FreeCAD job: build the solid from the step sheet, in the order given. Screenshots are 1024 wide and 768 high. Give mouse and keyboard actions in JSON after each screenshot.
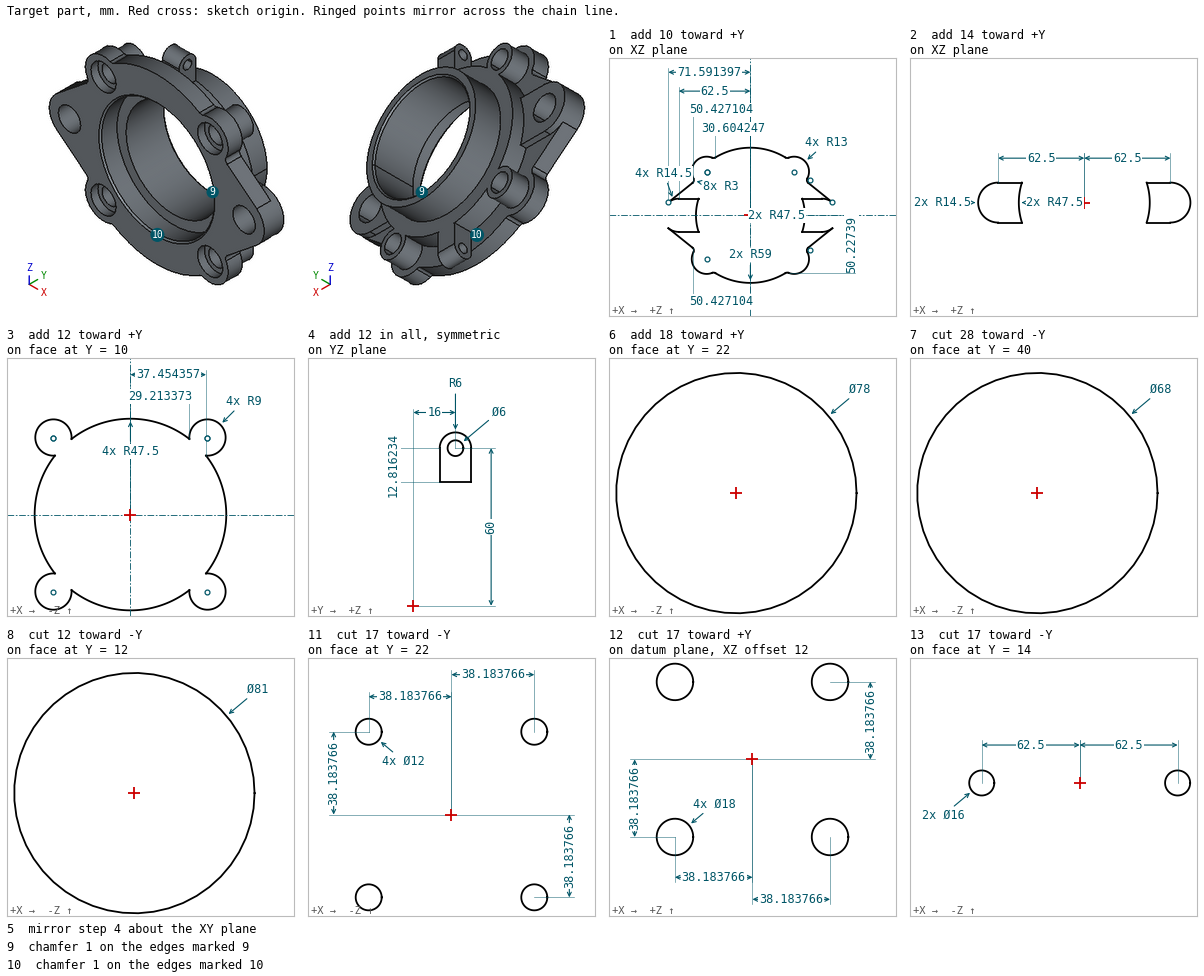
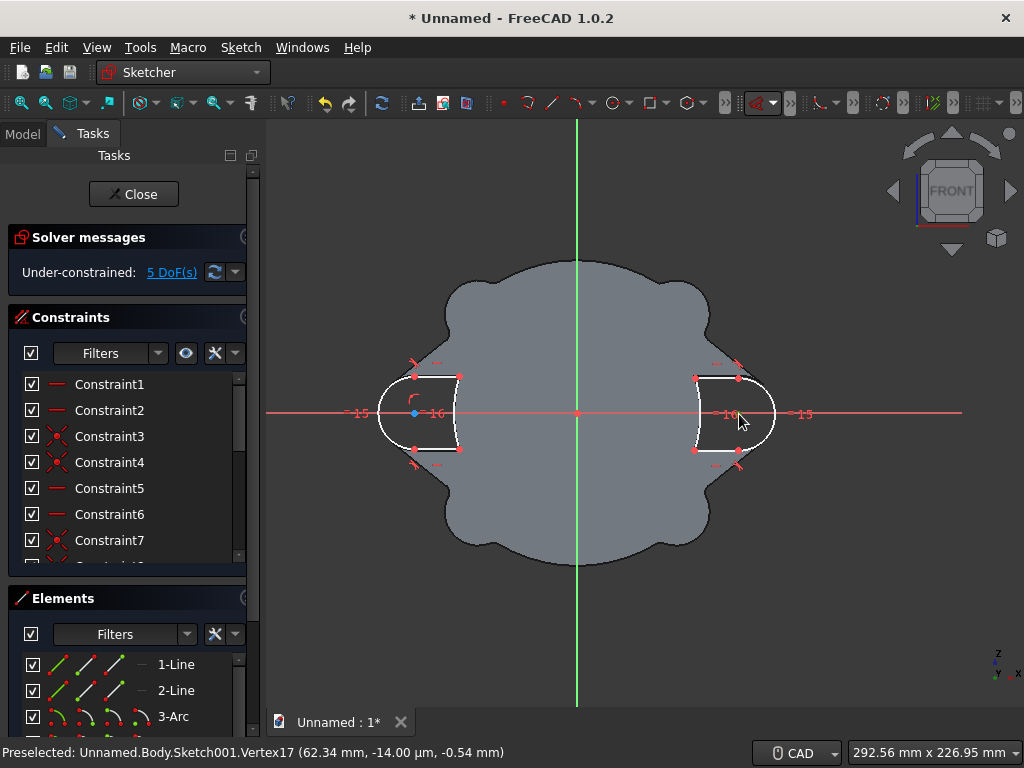
{"action": "left_click", "coordinate": [334, 413]}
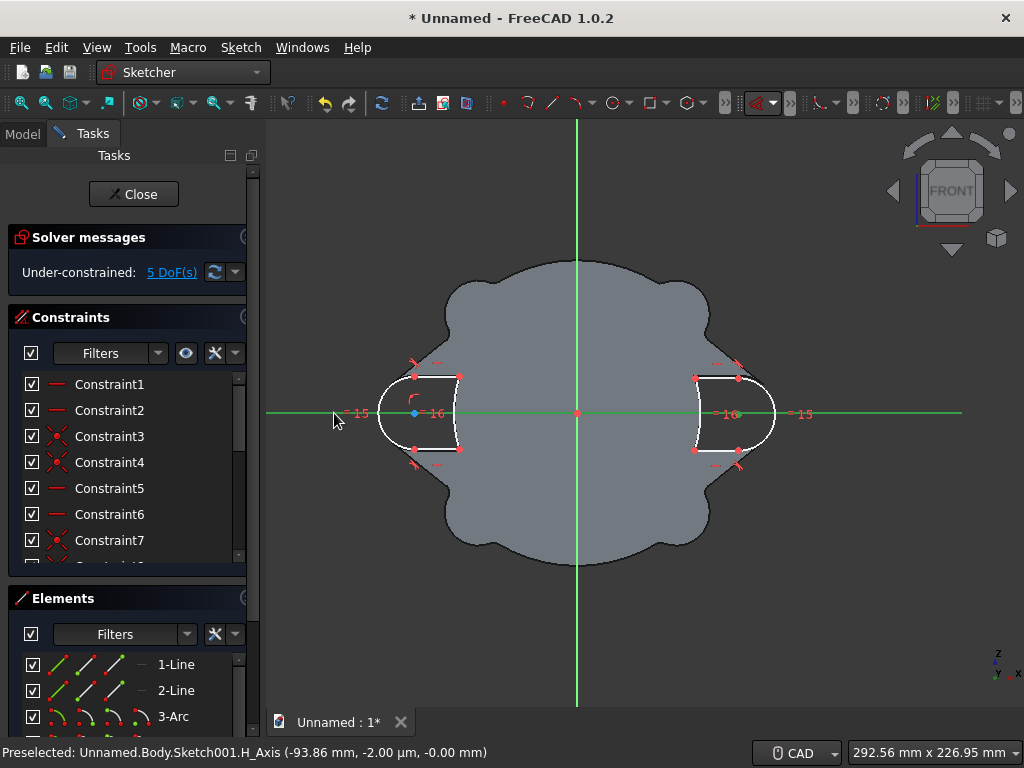
{"action": "key", "text": "c"}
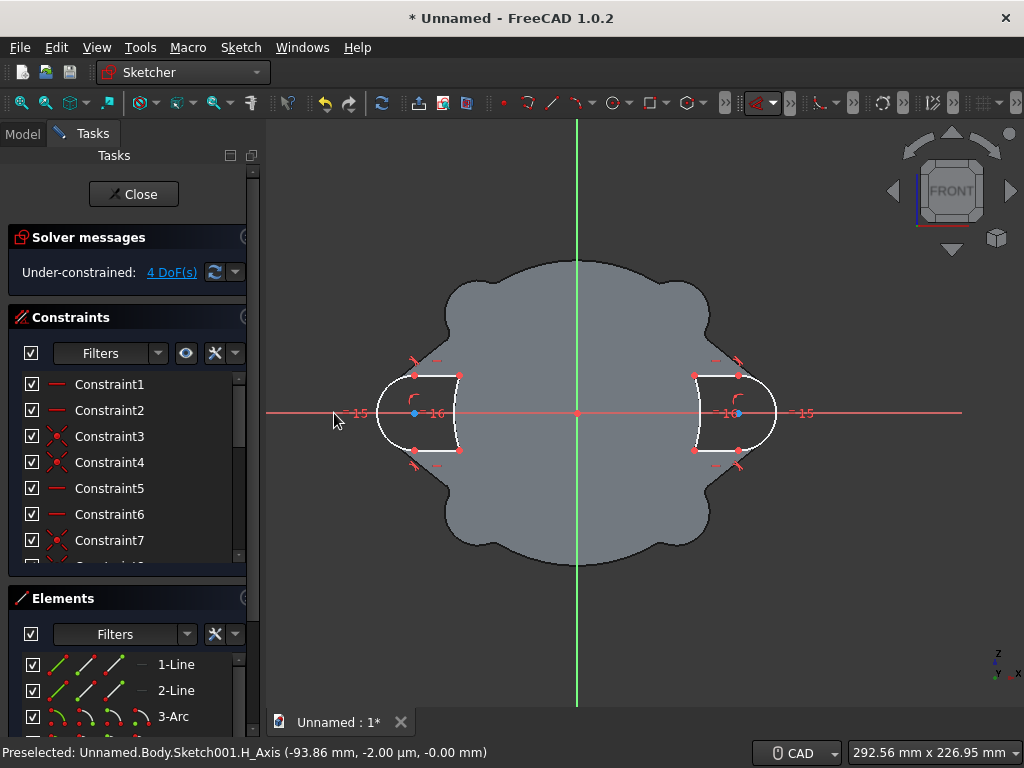
{"action": "key", "text": "d"}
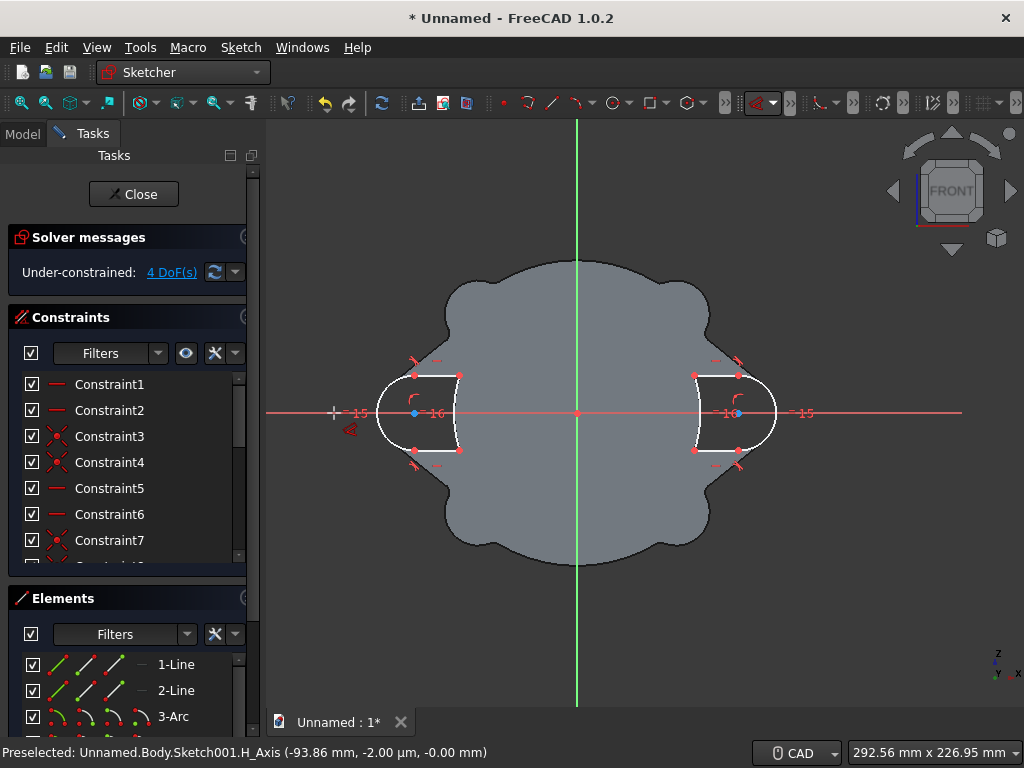
{"action": "left_click", "coordinate": [455, 398]}
{"action": "left_click", "coordinate": [423, 394]}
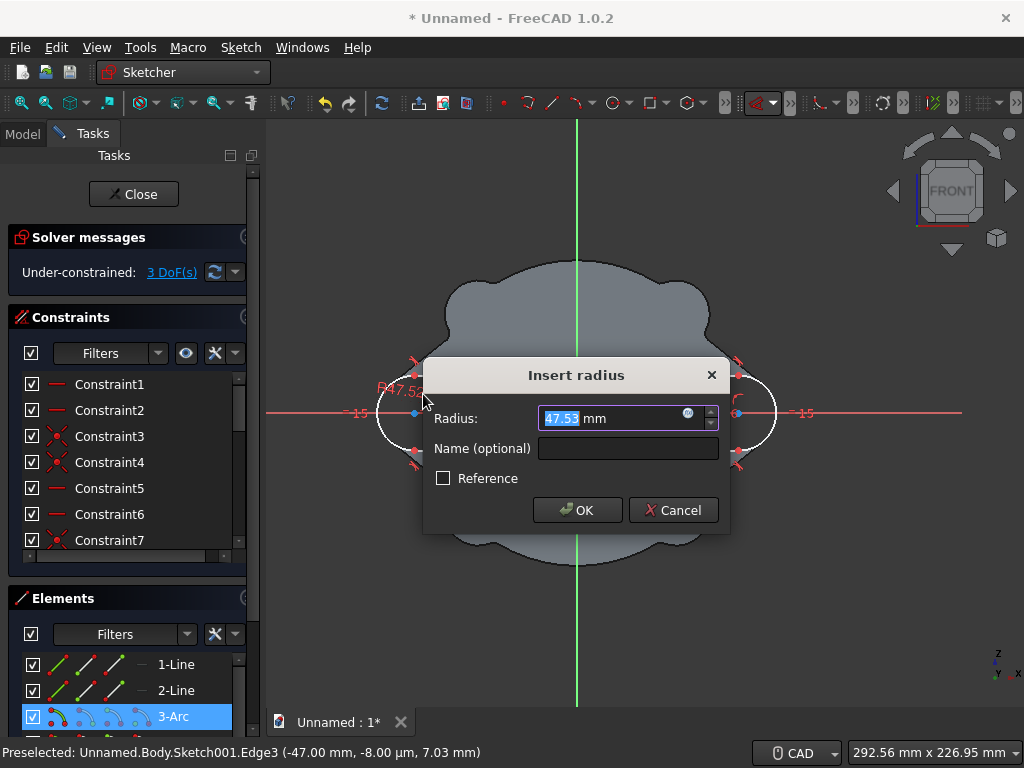
{"action": "type", "text": "47.5"}
{"action": "key", "text": "Return"}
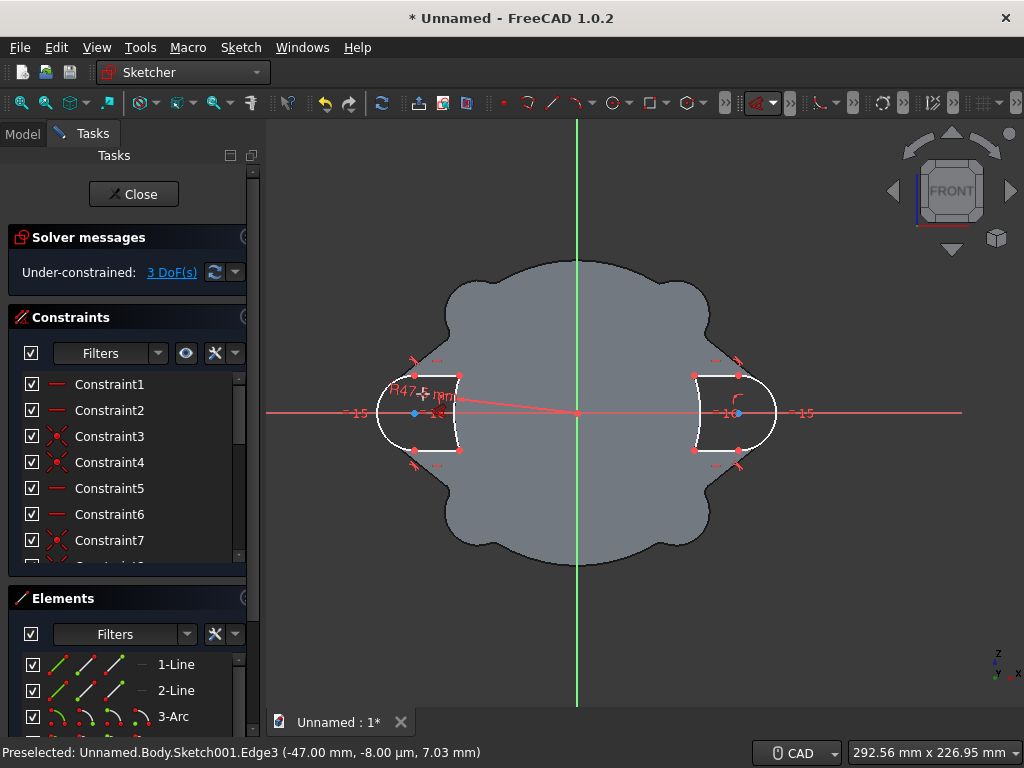
{"action": "left_click", "coordinate": [384, 391]}
{"action": "left_click", "coordinate": [358, 372]}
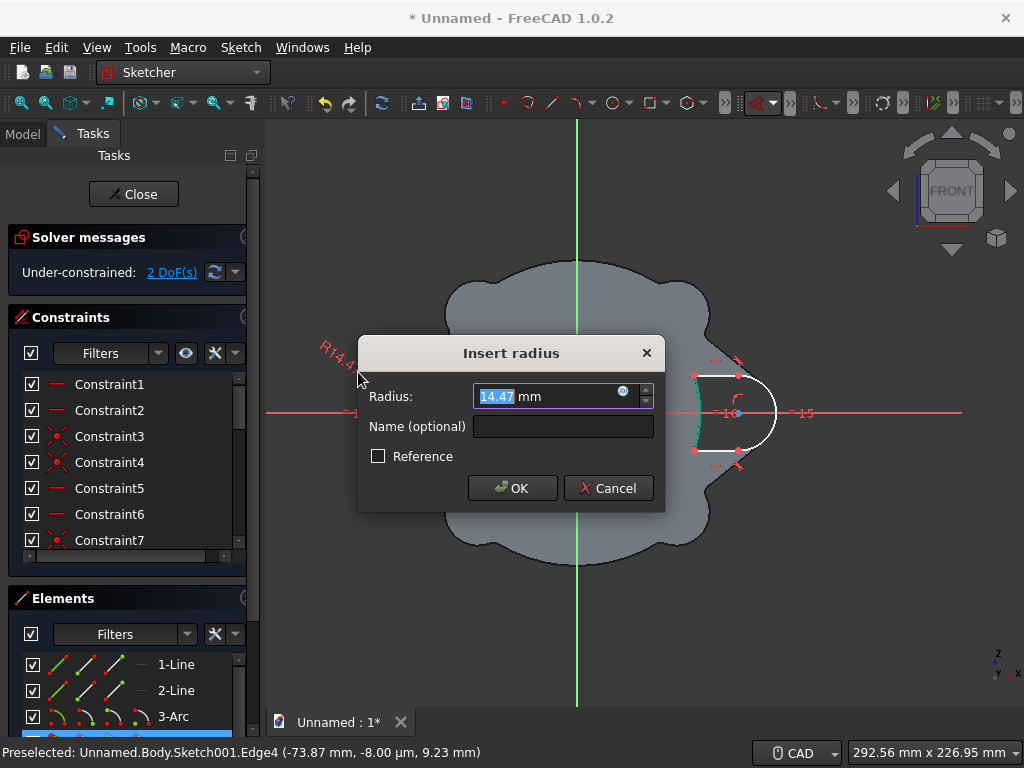
{"action": "type", "text": "14.5"}
{"action": "key", "text": "Return"}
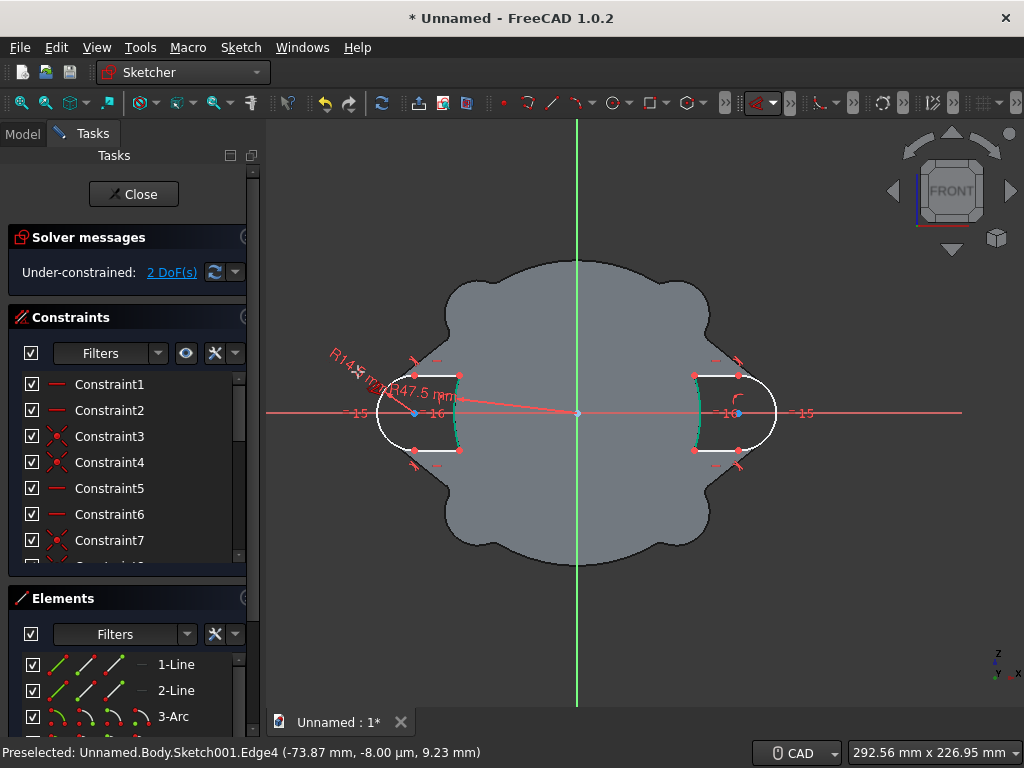
{"action": "left_click", "coordinate": [415, 376]}
{"action": "left_click", "coordinate": [496, 342]}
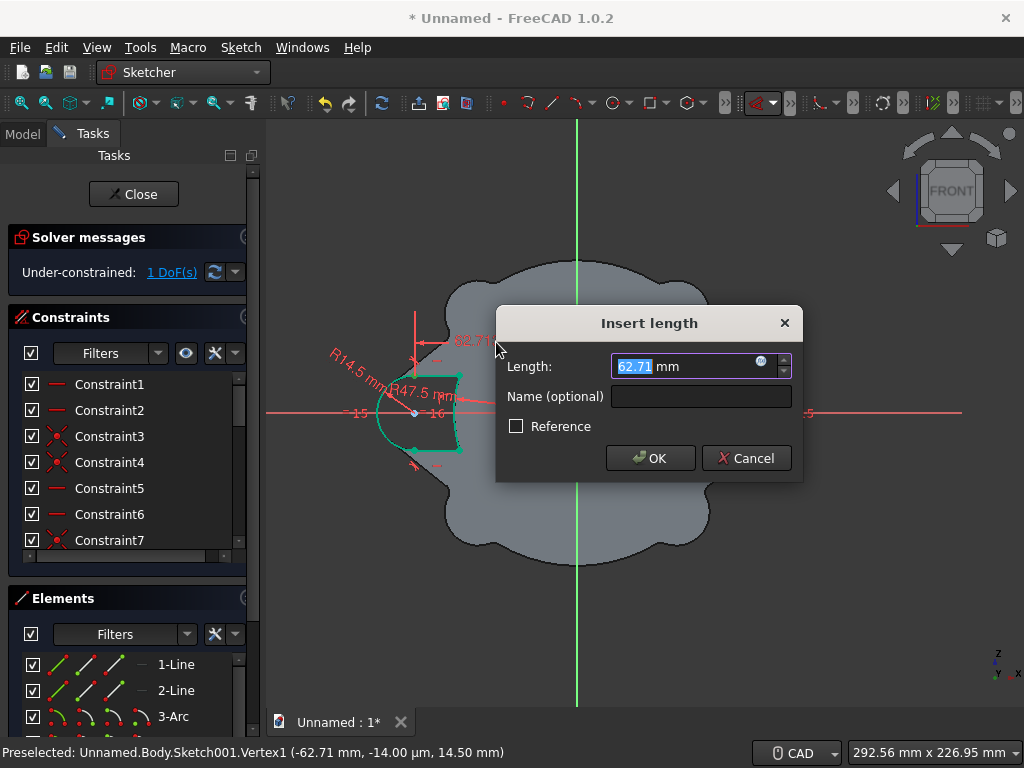
{"action": "type", "text": "62.5"}
{"action": "key", "text": "Return"}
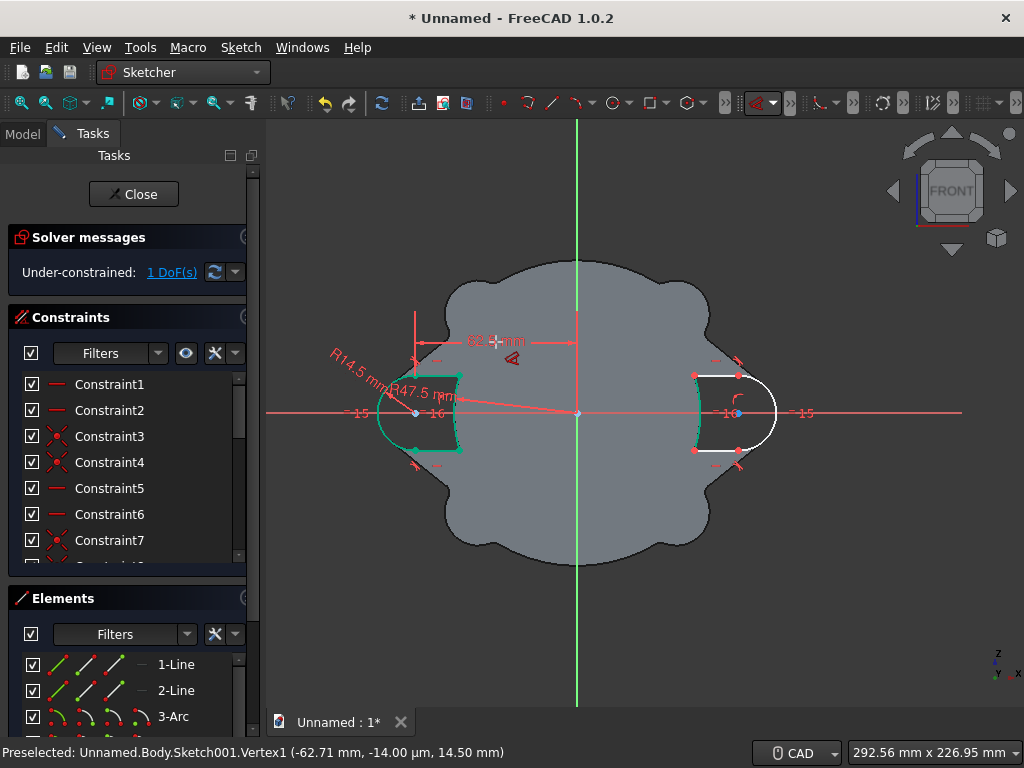
{"action": "left_click", "coordinate": [739, 376]}
{"action": "left_click", "coordinate": [658, 342]}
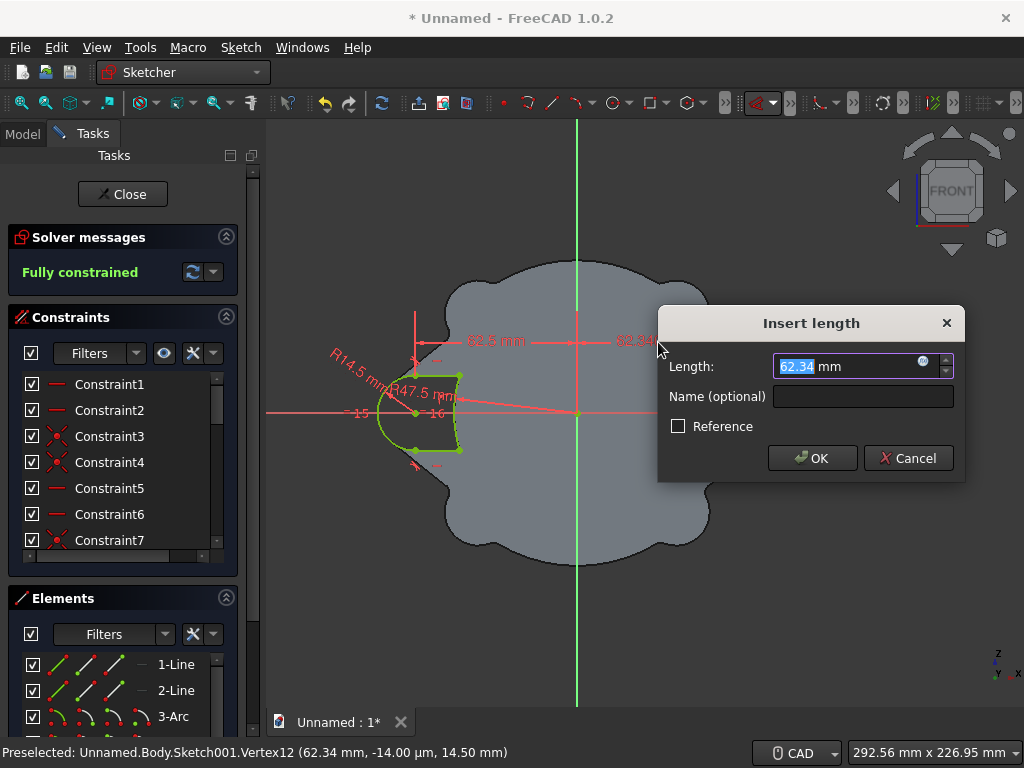
{"action": "type", "text": "62.5"}
{"action": "key", "text": "Return"}
{"action": "key", "text": "Escape"}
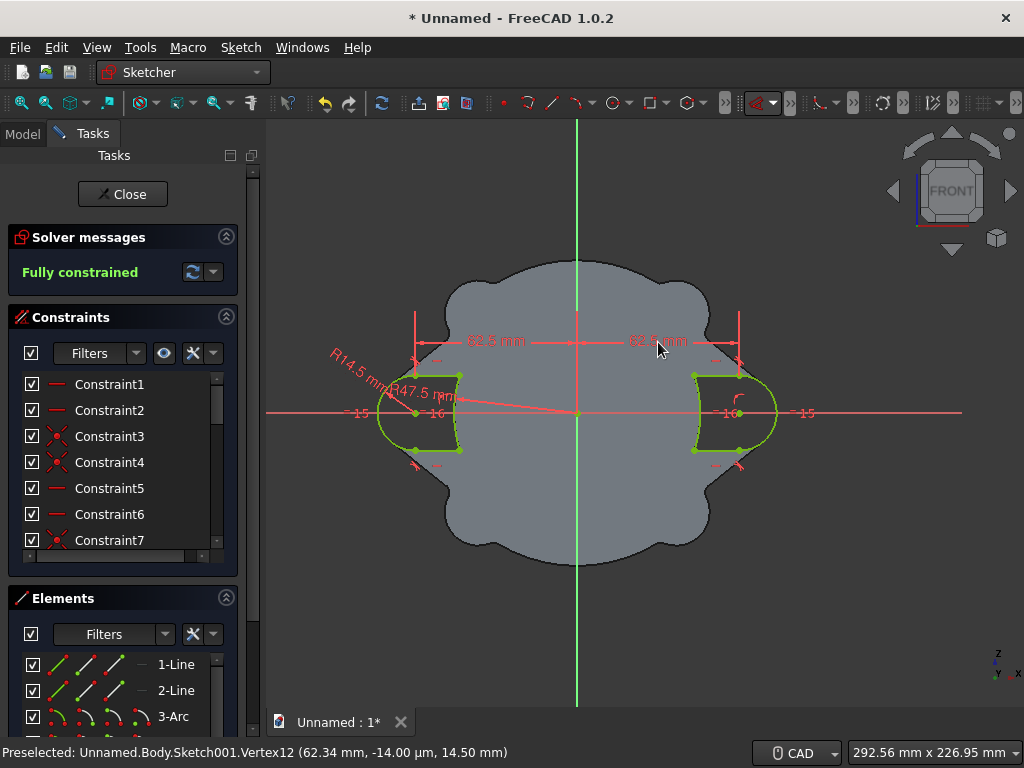
{"action": "left_click", "coordinate": [123, 194]}